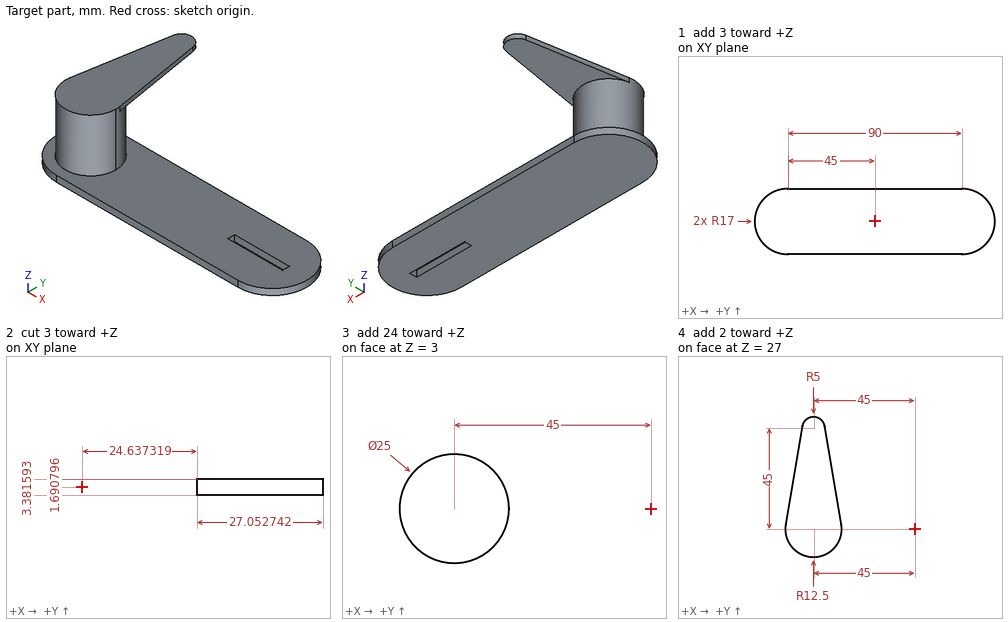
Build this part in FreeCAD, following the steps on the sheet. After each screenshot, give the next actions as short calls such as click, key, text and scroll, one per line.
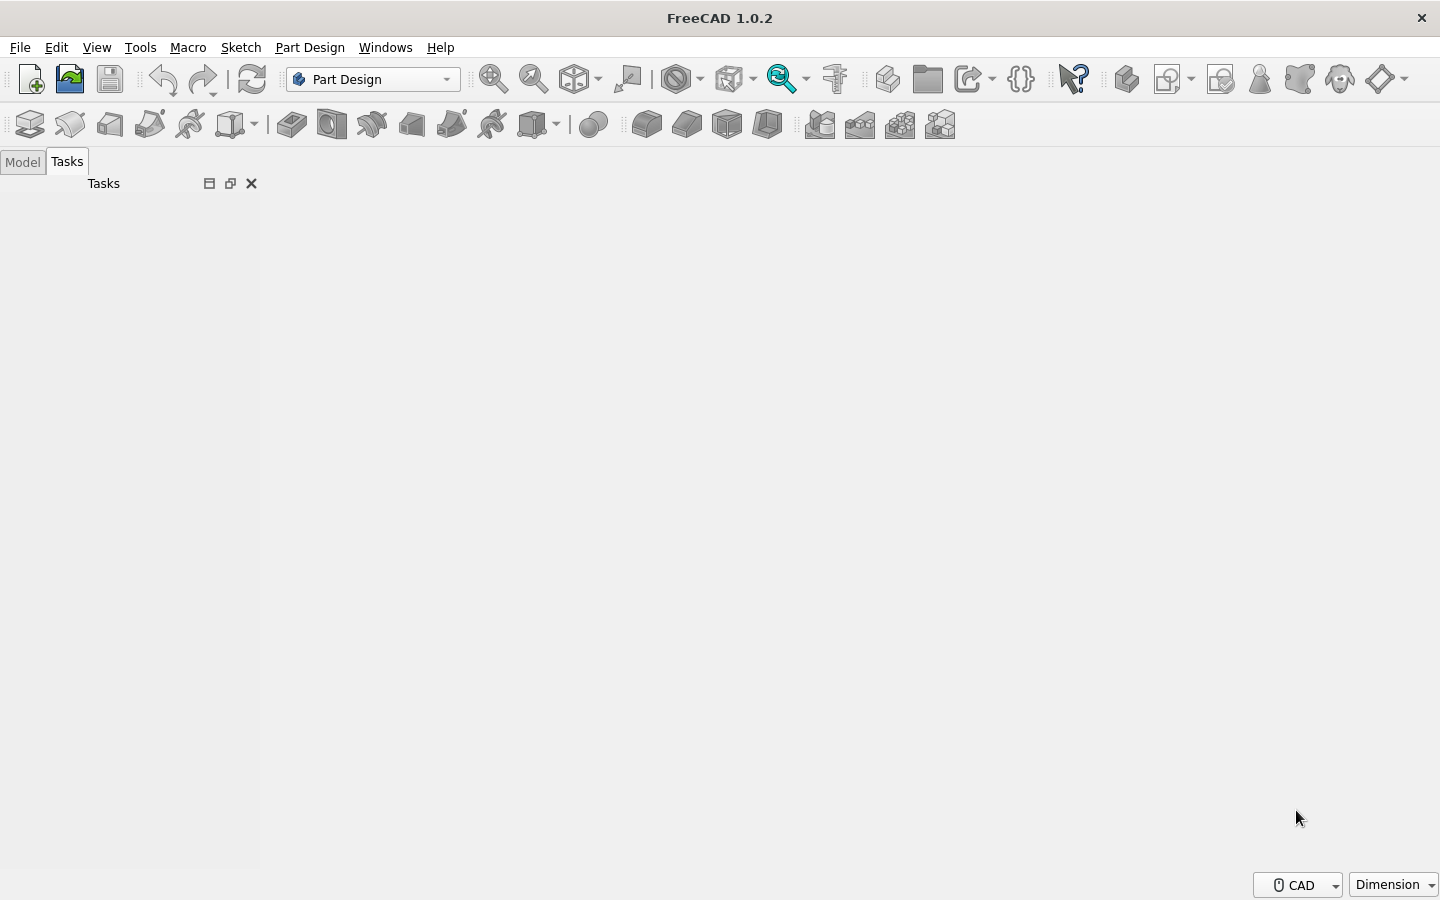
click(30, 80)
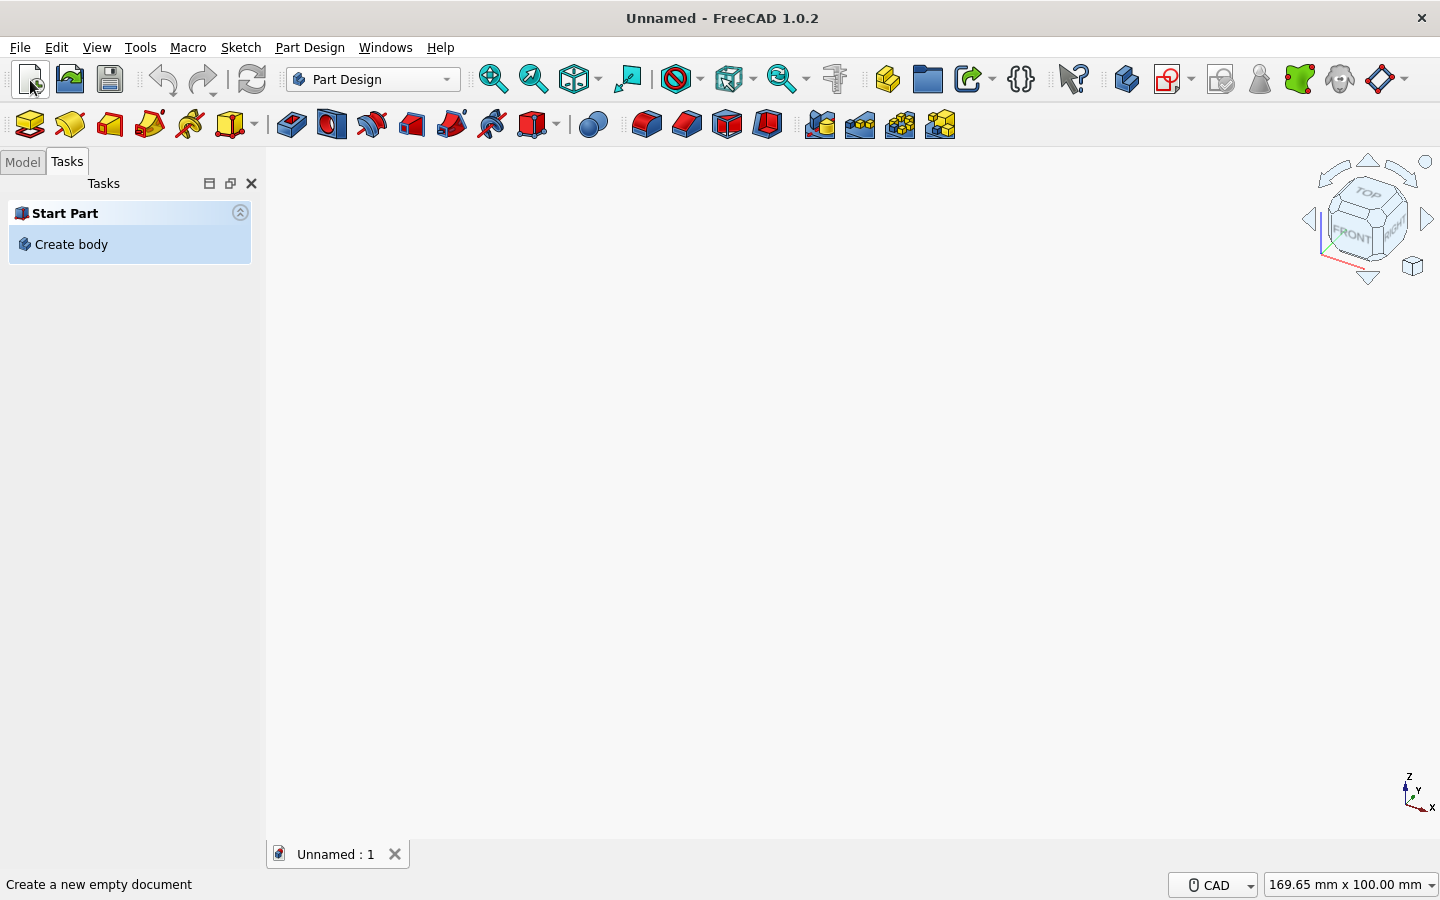
click(1168, 80)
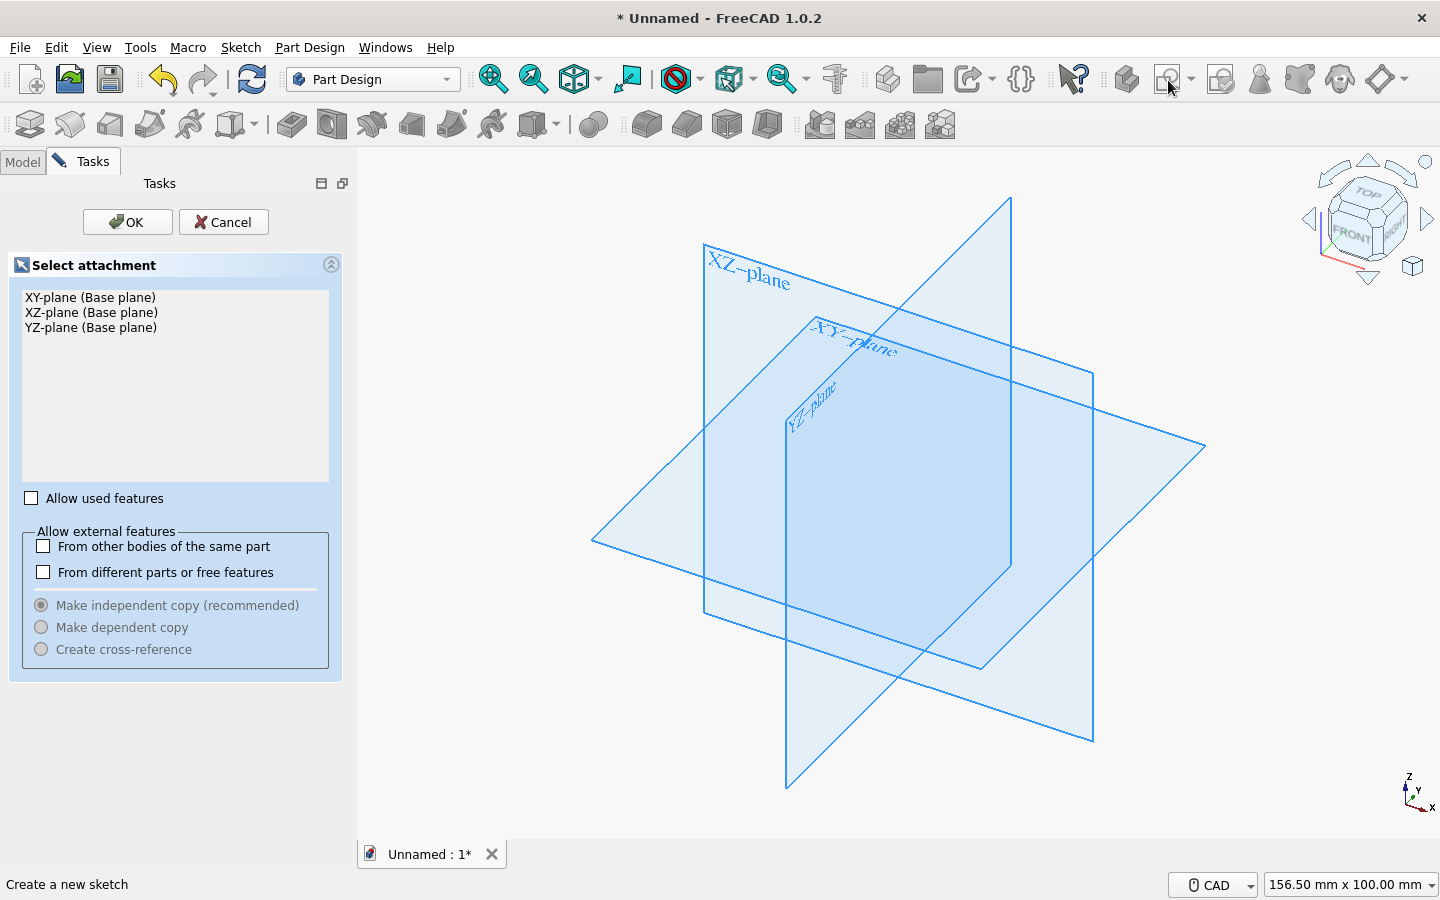
click(82, 298)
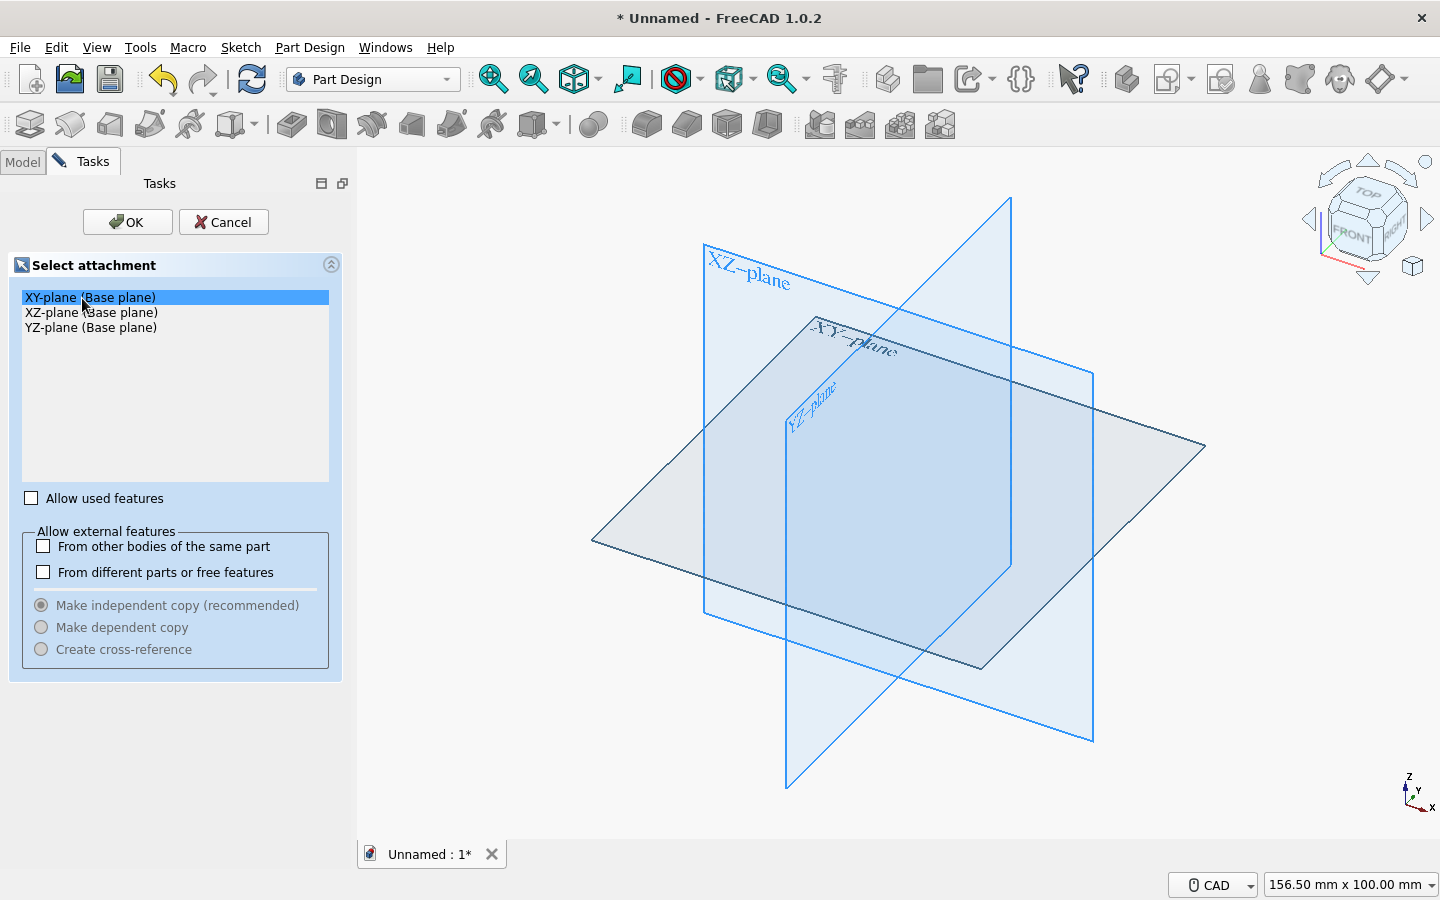
click(128, 222)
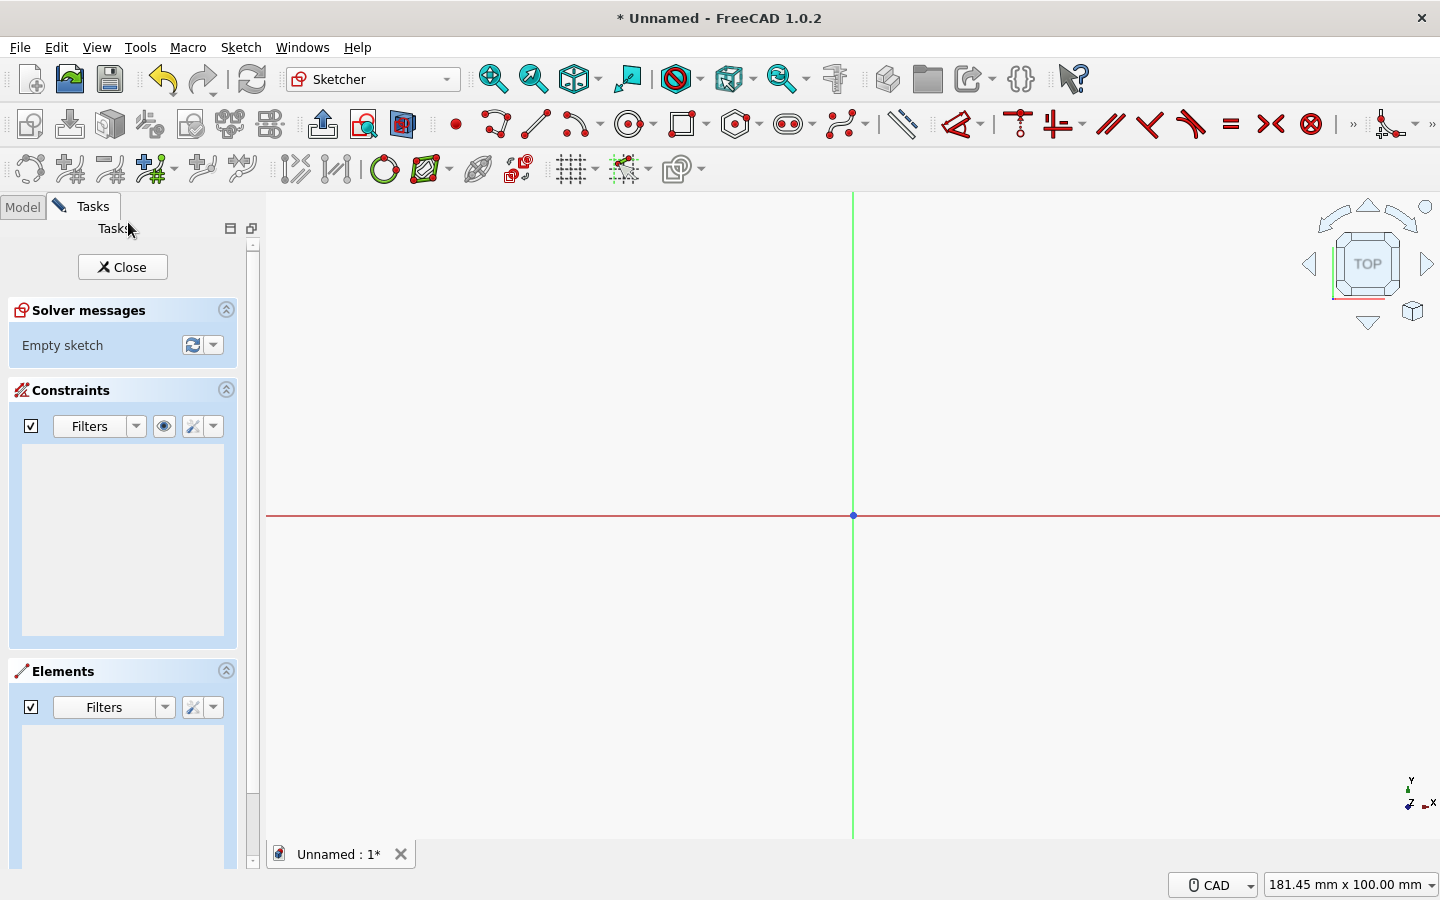
scroll(475, 516, down, 1)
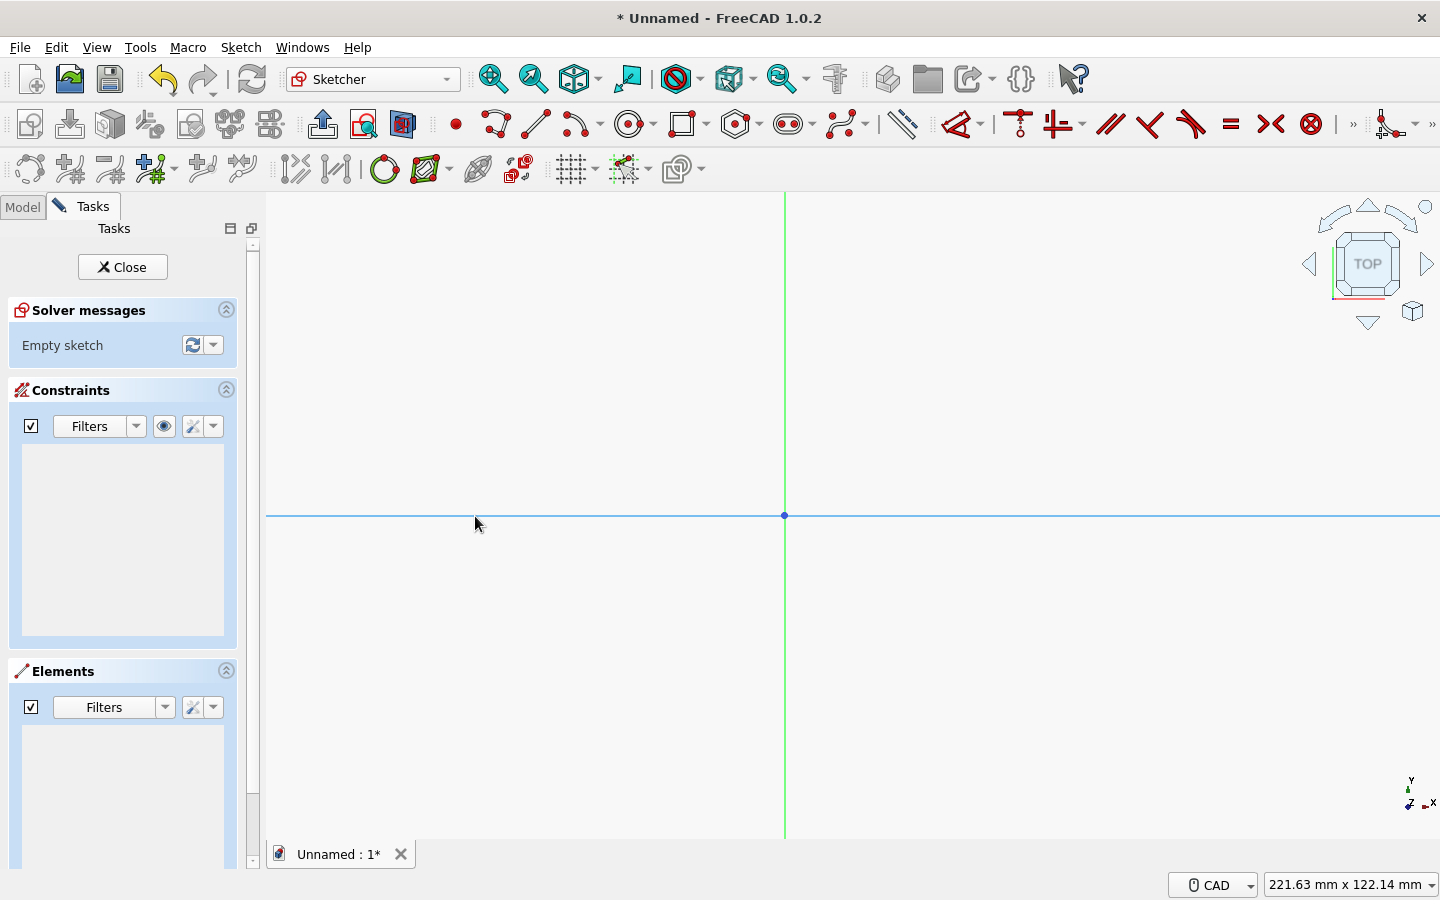
click(788, 124)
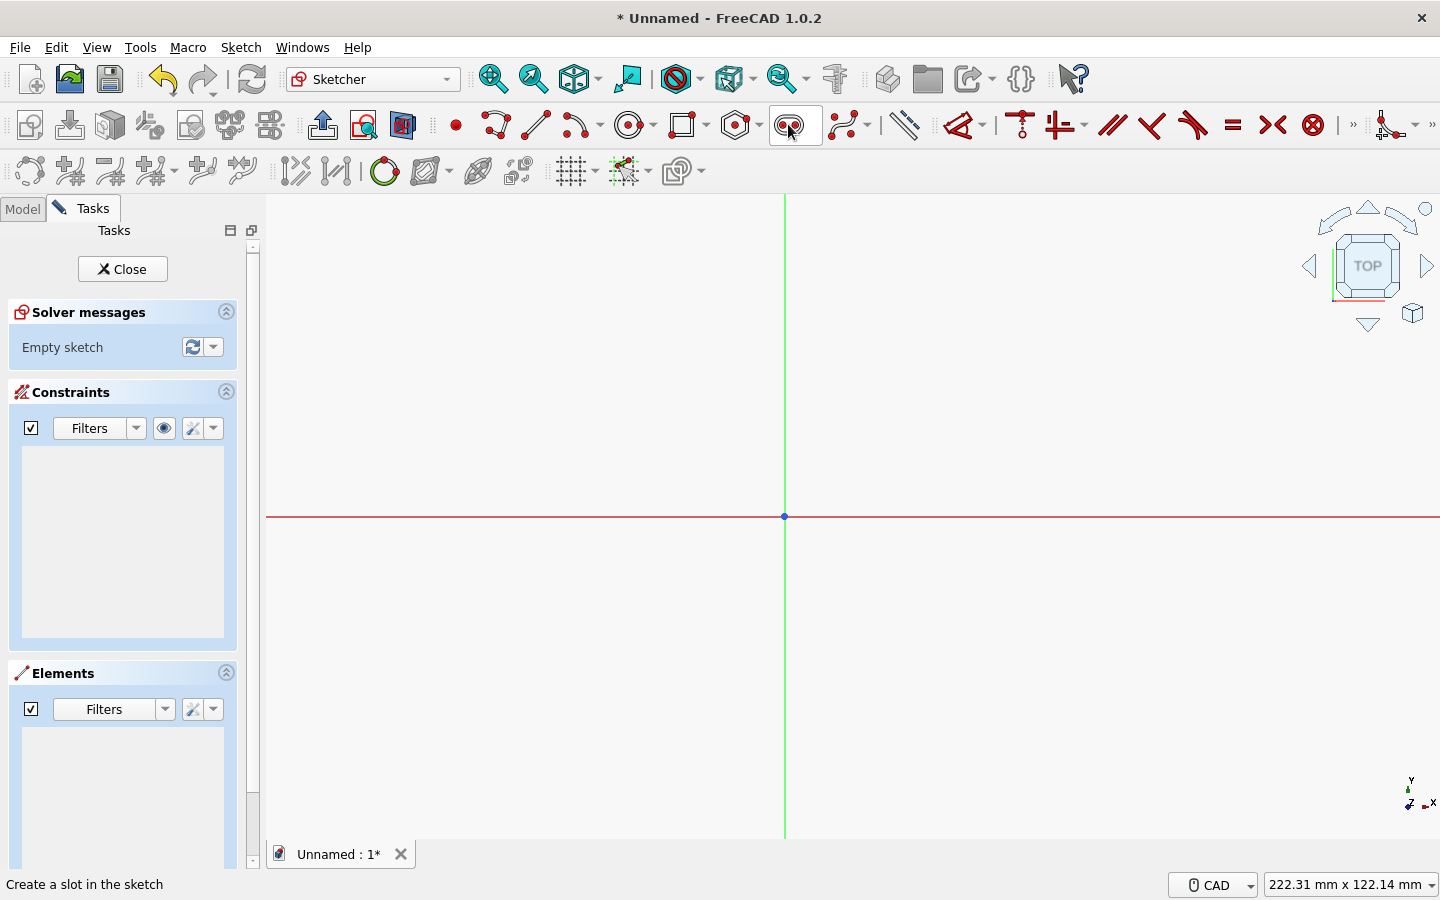
click(547, 517)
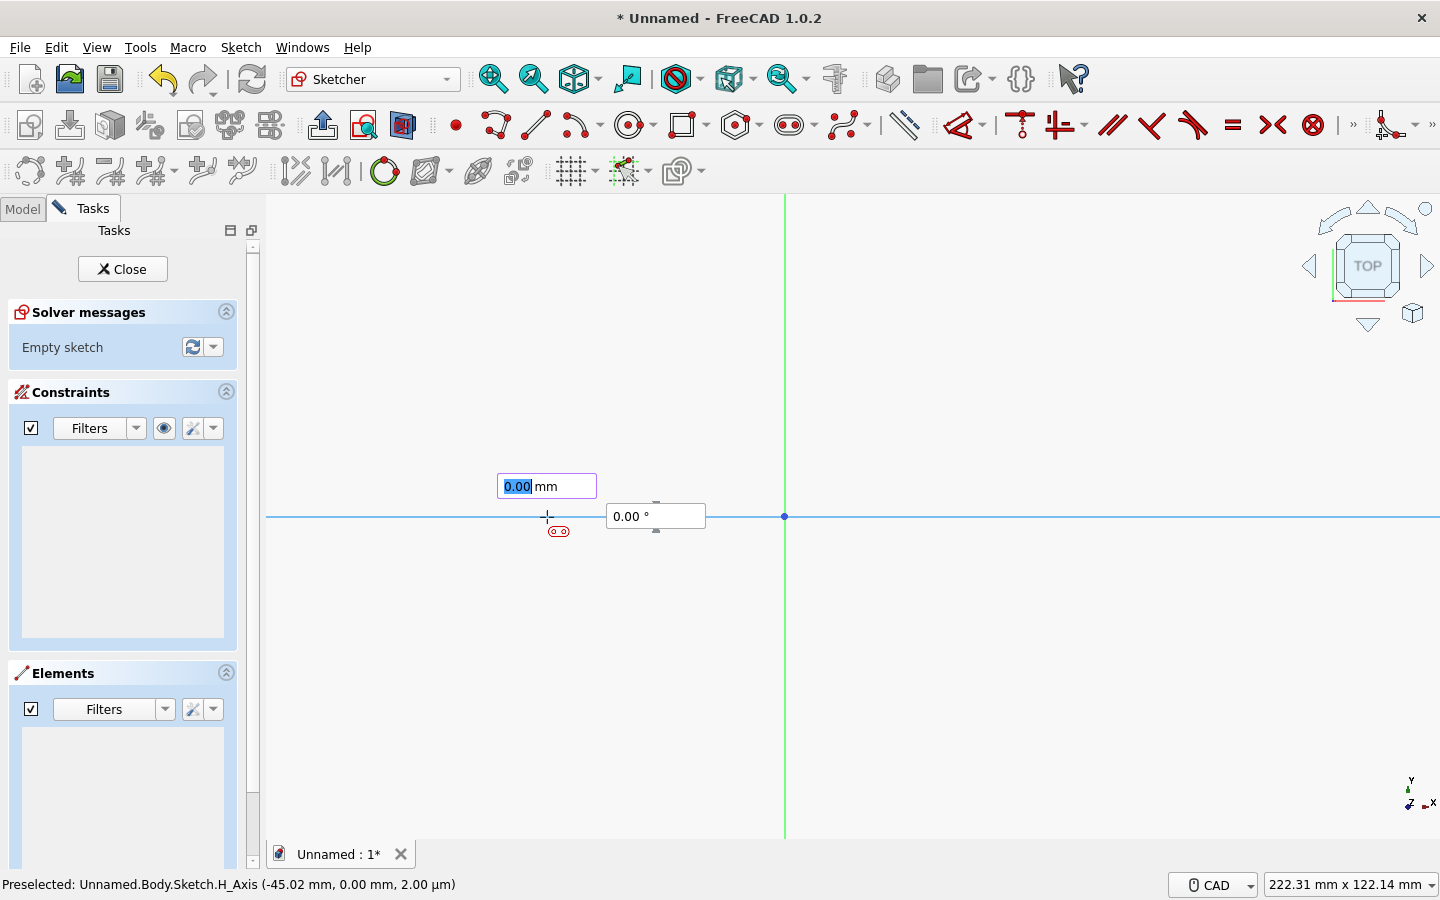
click(1022, 508)